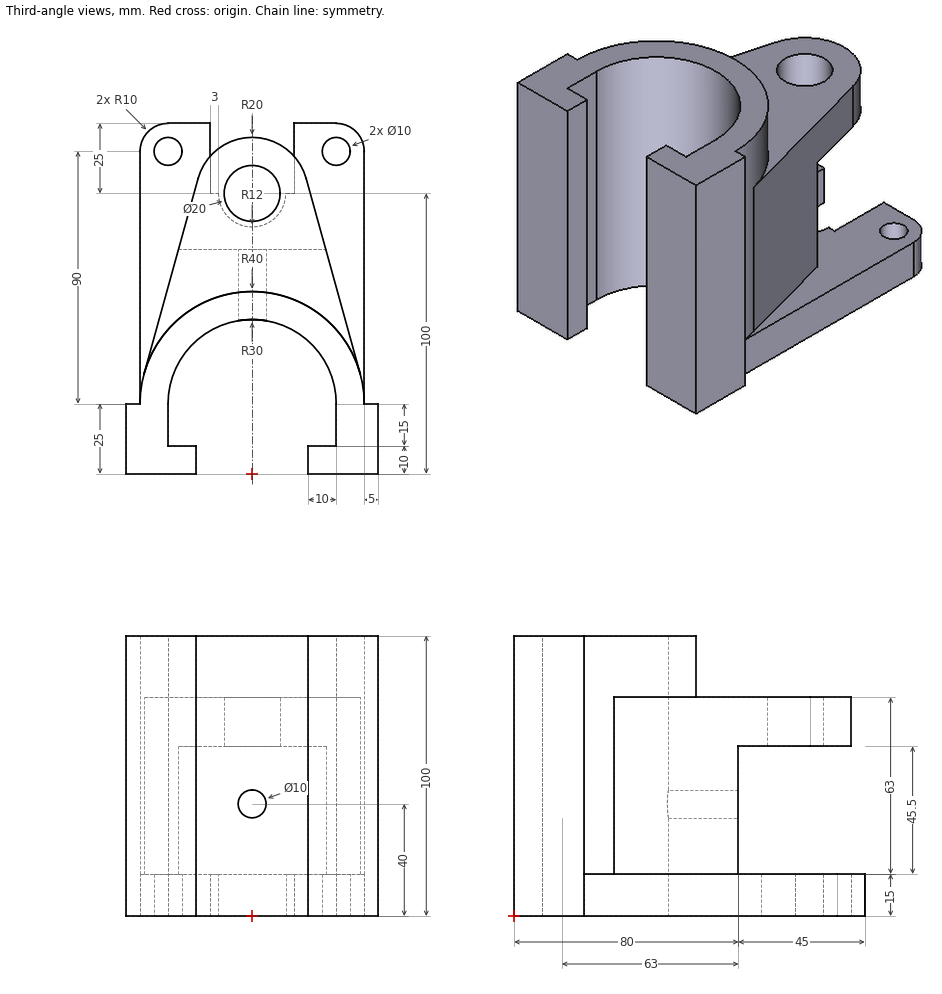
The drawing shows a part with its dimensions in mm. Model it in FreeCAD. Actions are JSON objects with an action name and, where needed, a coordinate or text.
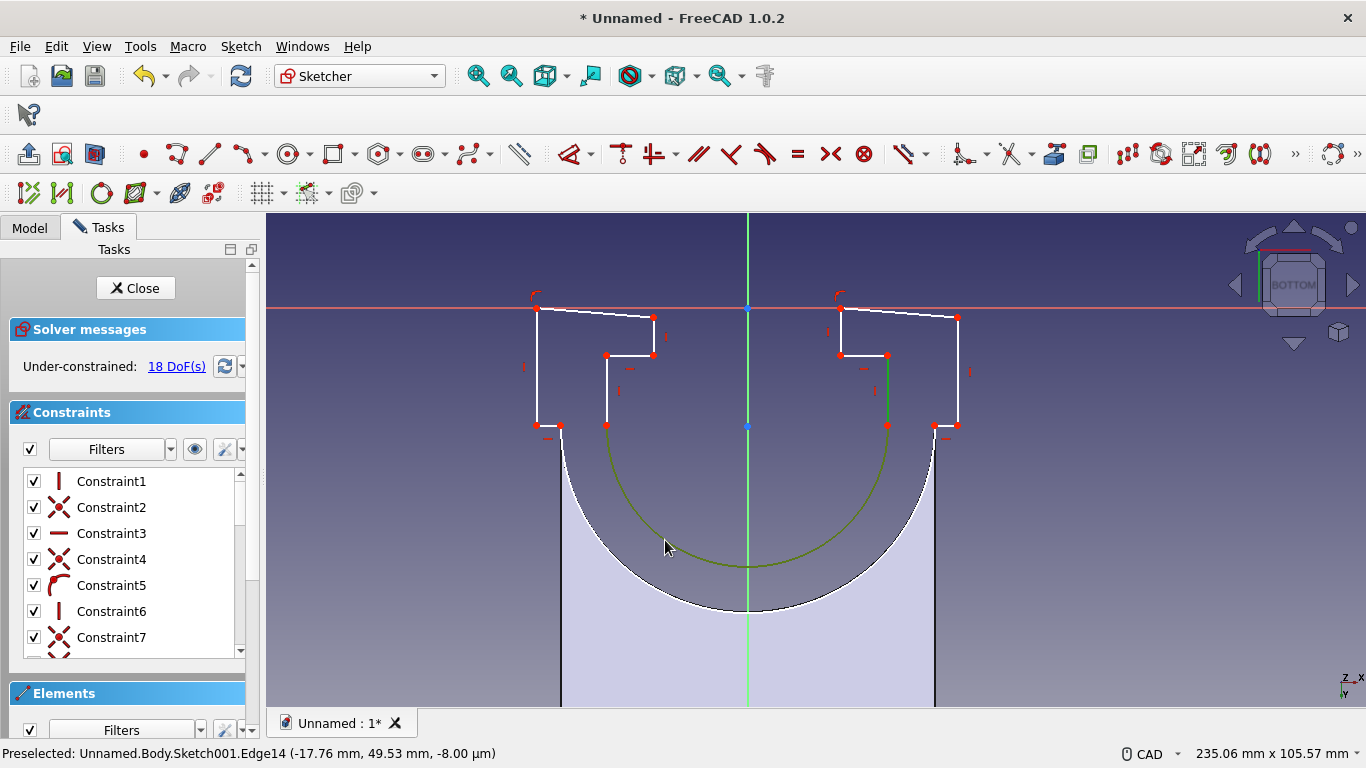
{"action": "key", "text": "t"}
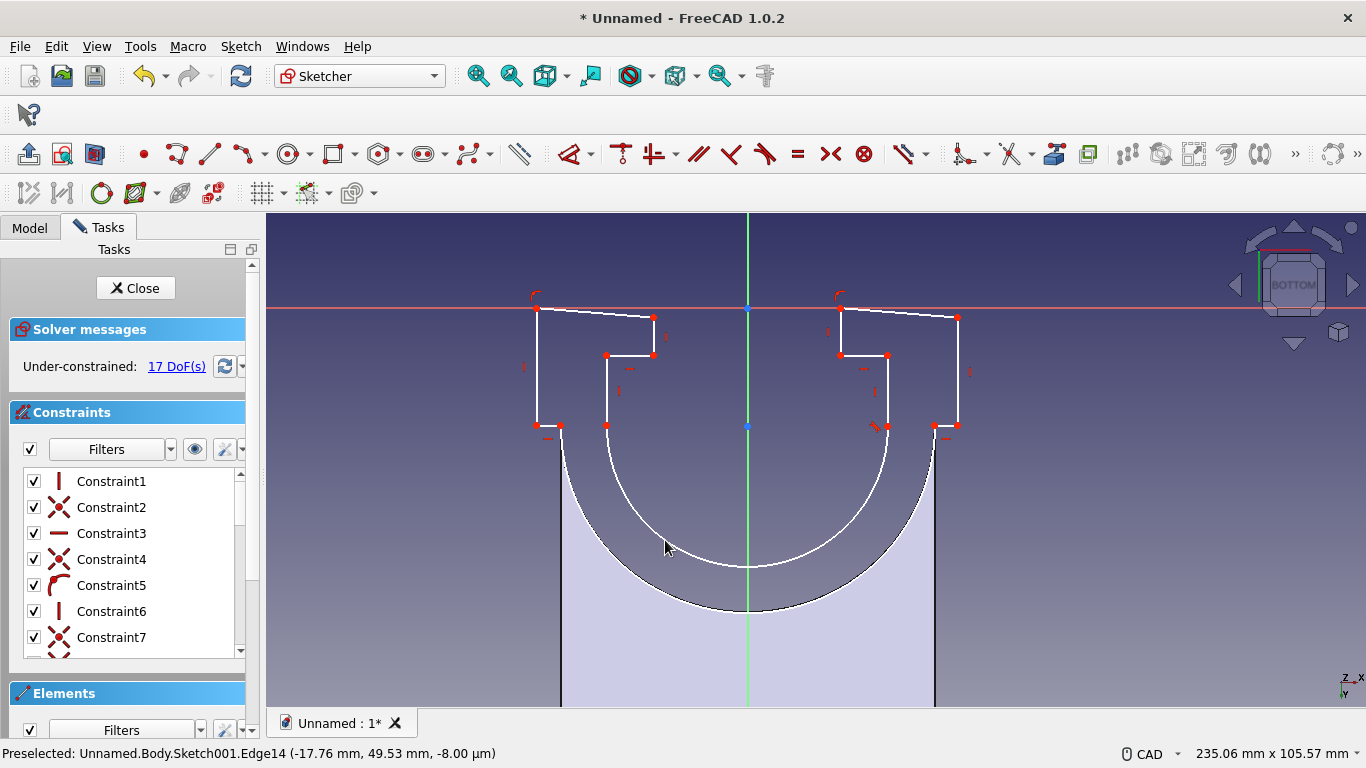
{"action": "left_click", "coordinate": [607, 377]}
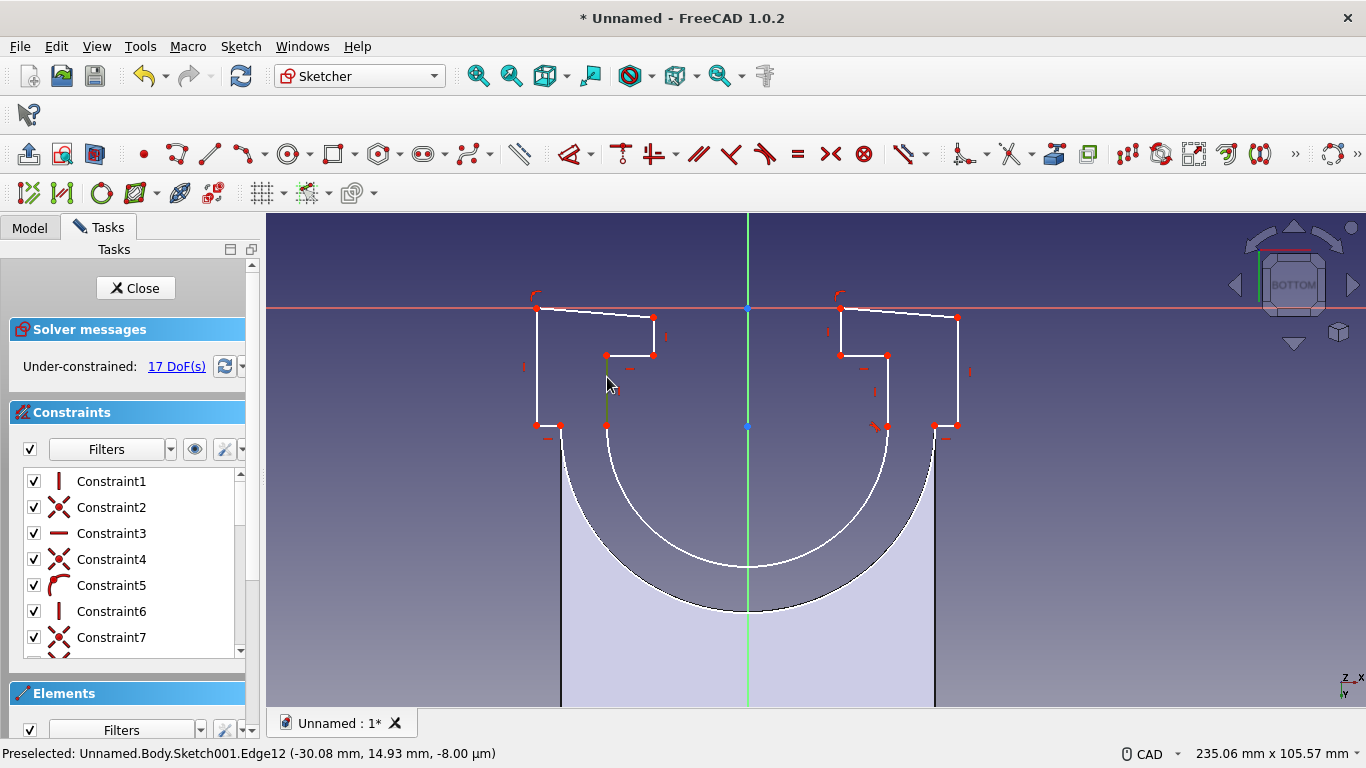
{"action": "left_click", "coordinate": [664, 540]}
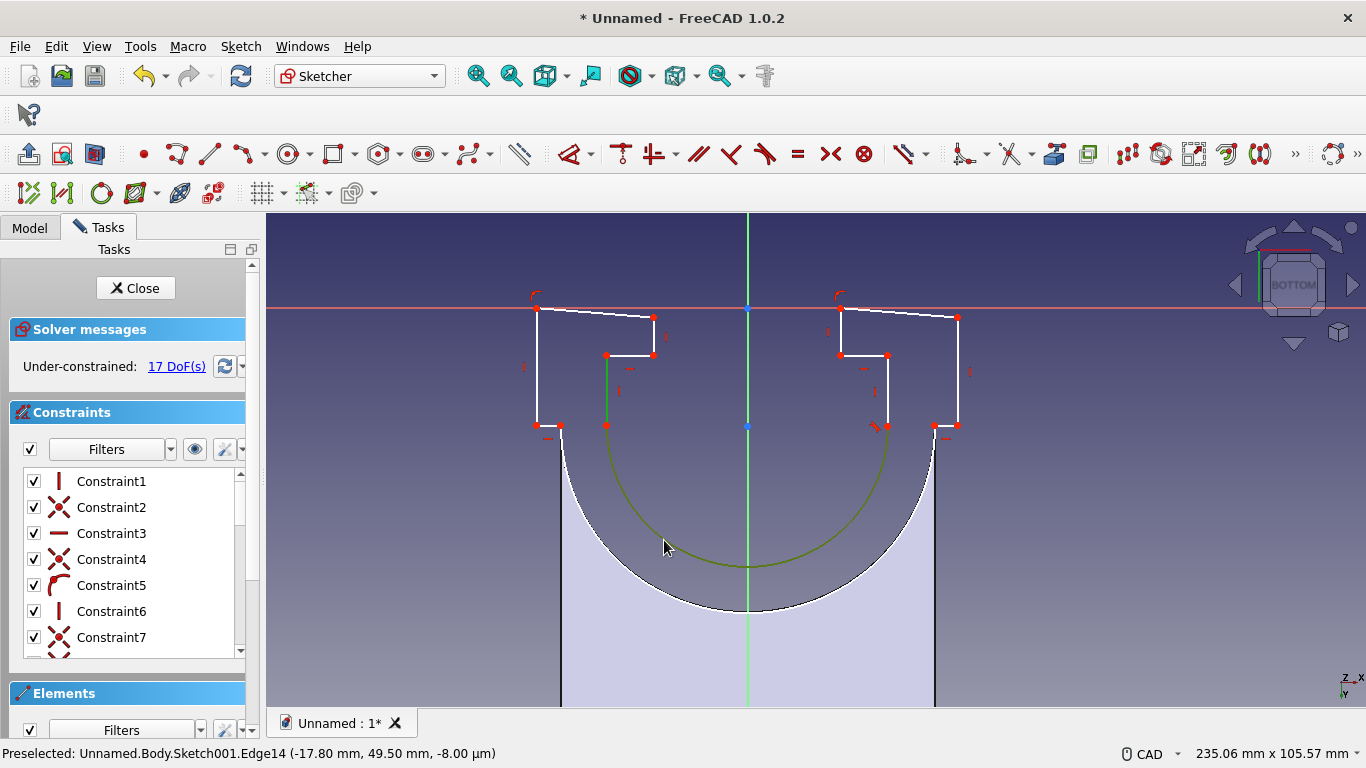
{"action": "key", "text": "t"}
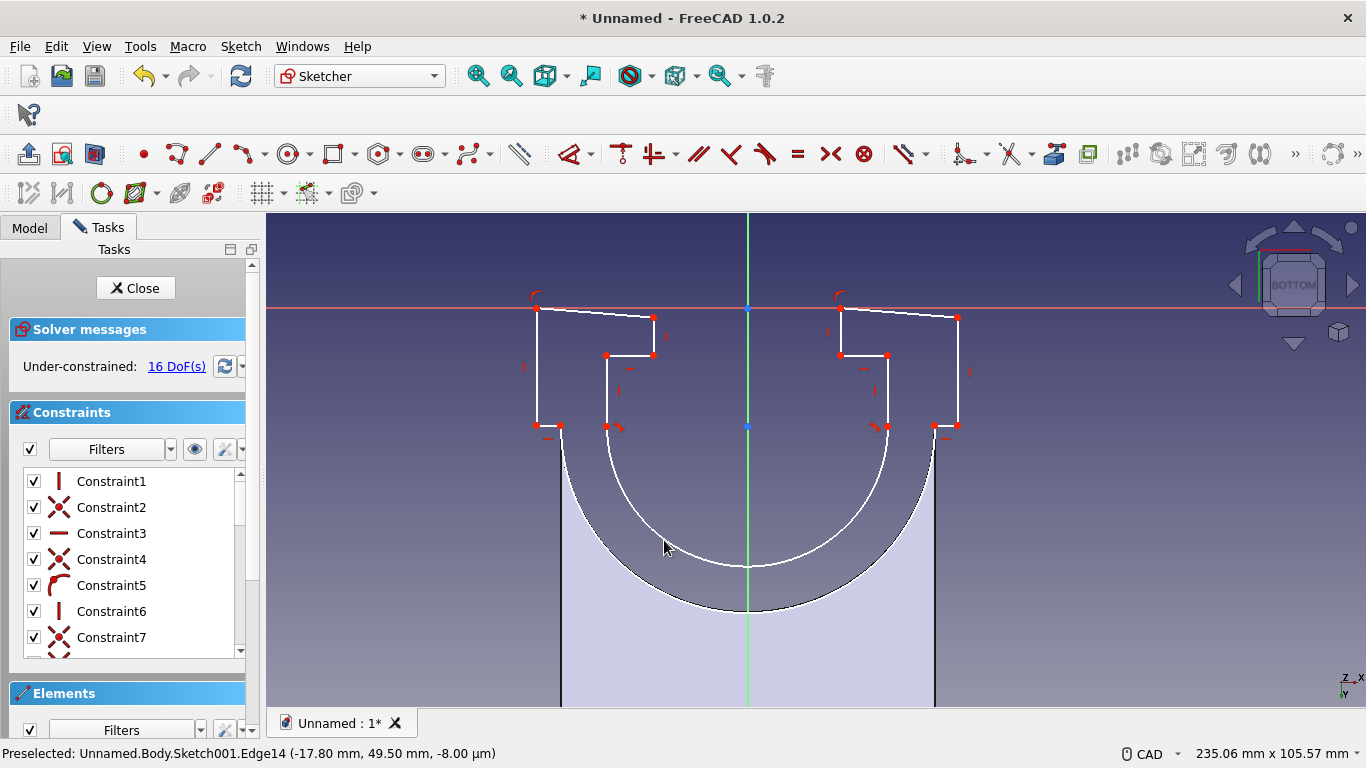
{"action": "left_click", "coordinate": [876, 311]}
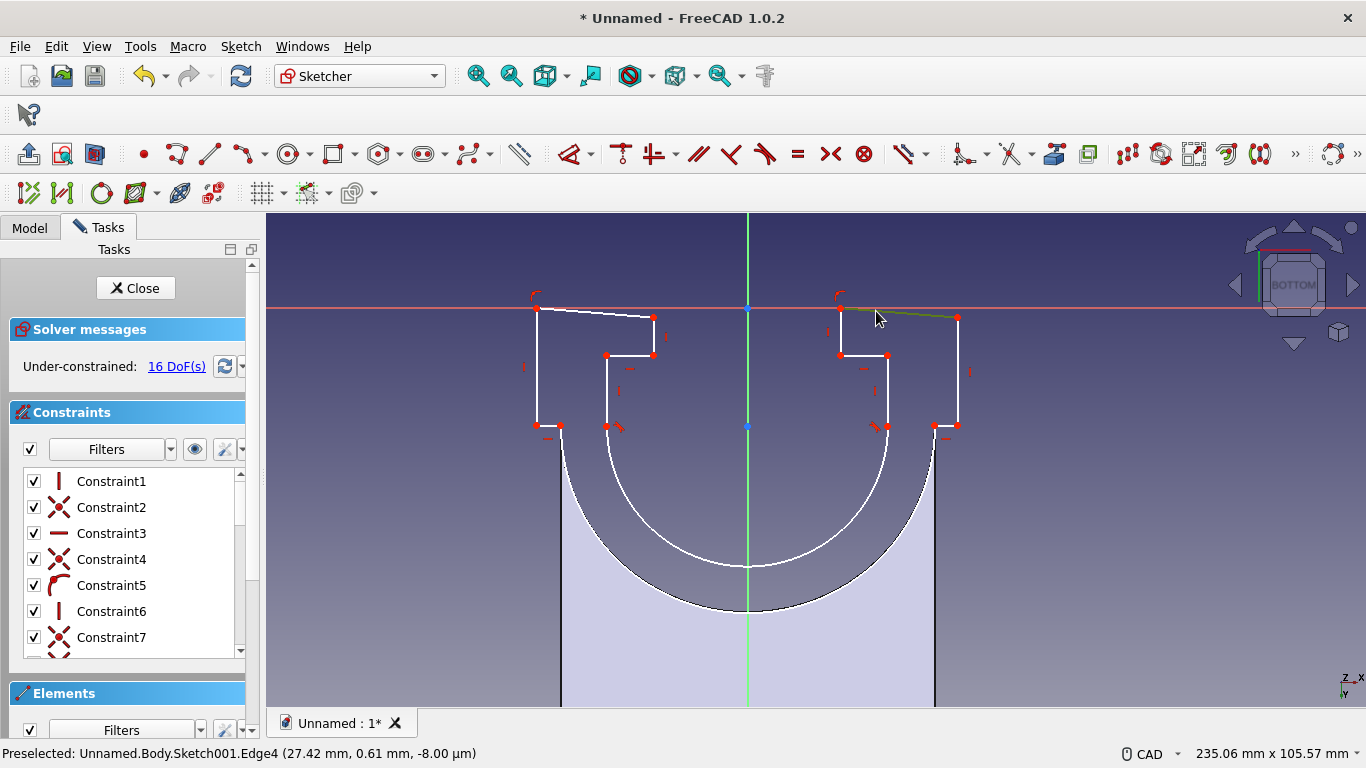
{"action": "key", "text": "h"}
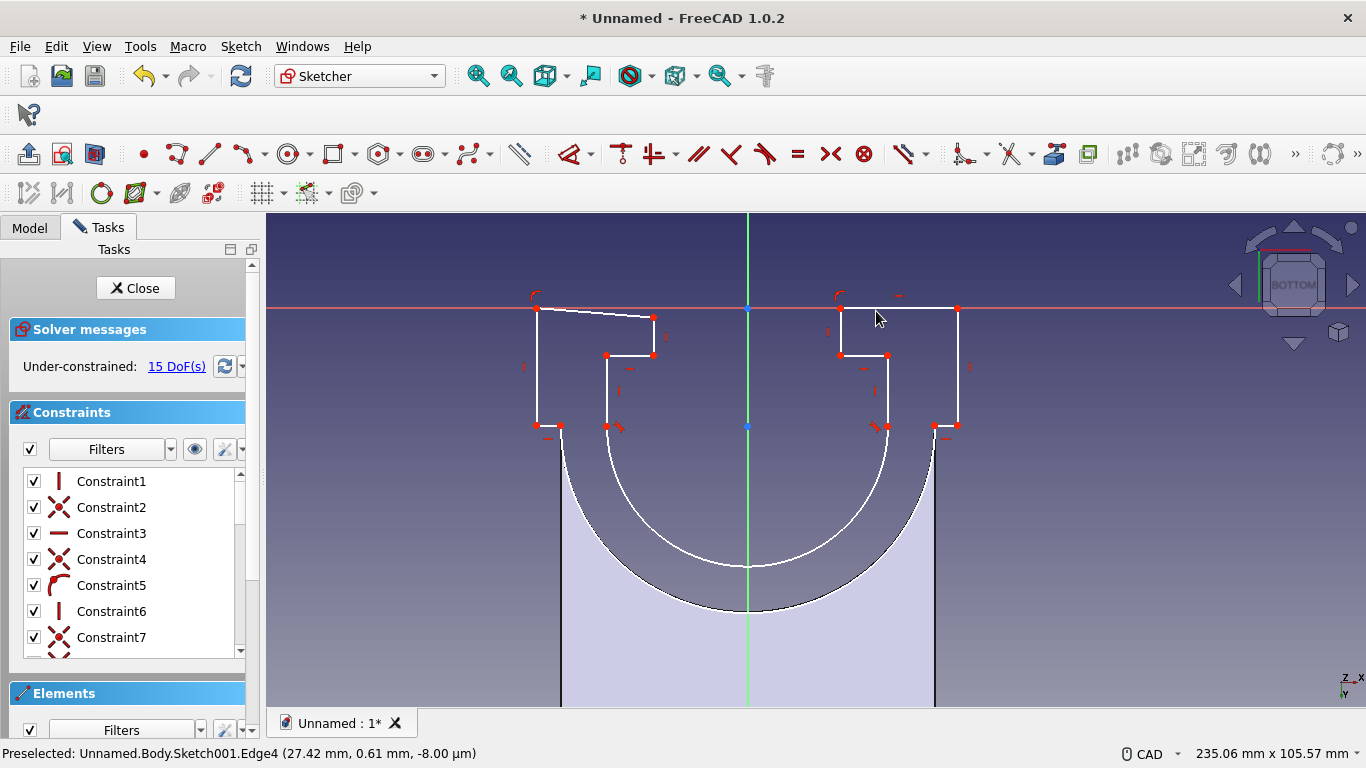
{"action": "left_click", "coordinate": [572, 311]}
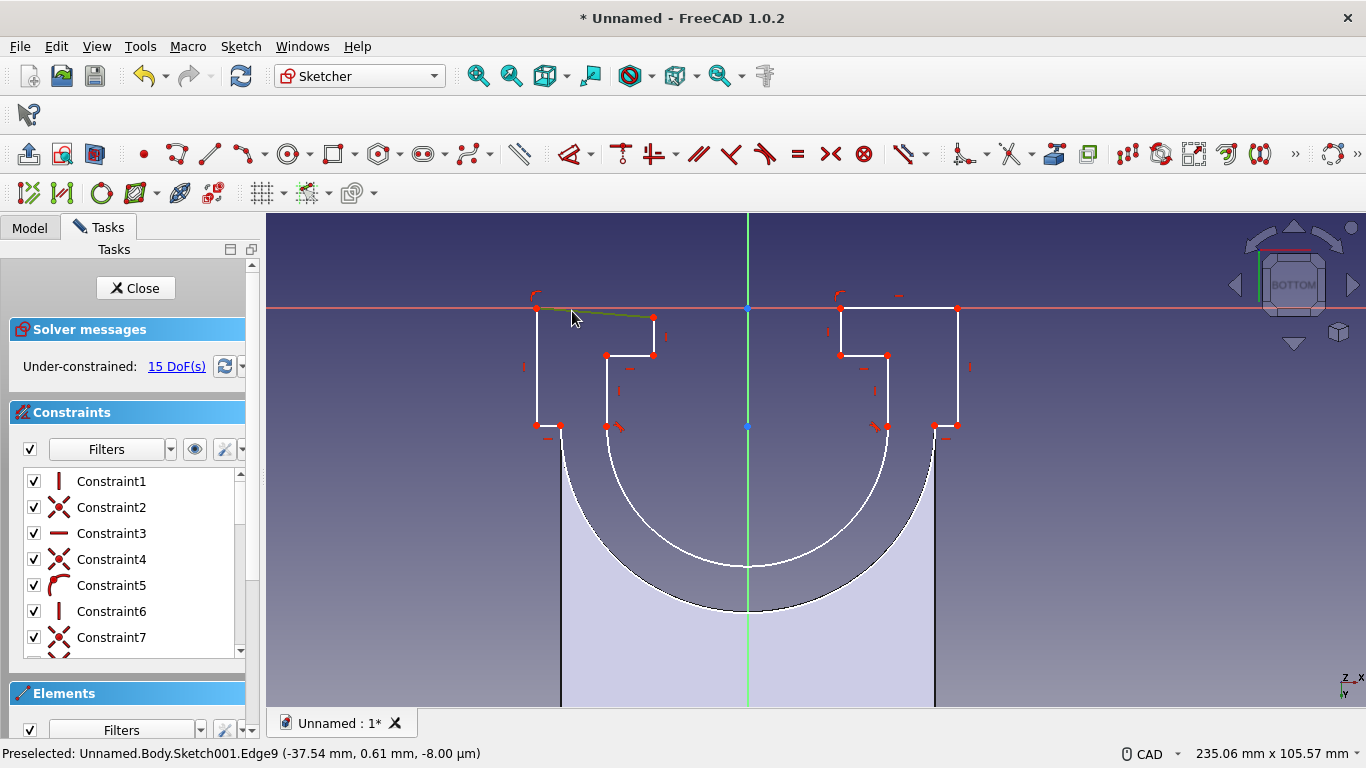
{"action": "key", "text": "h"}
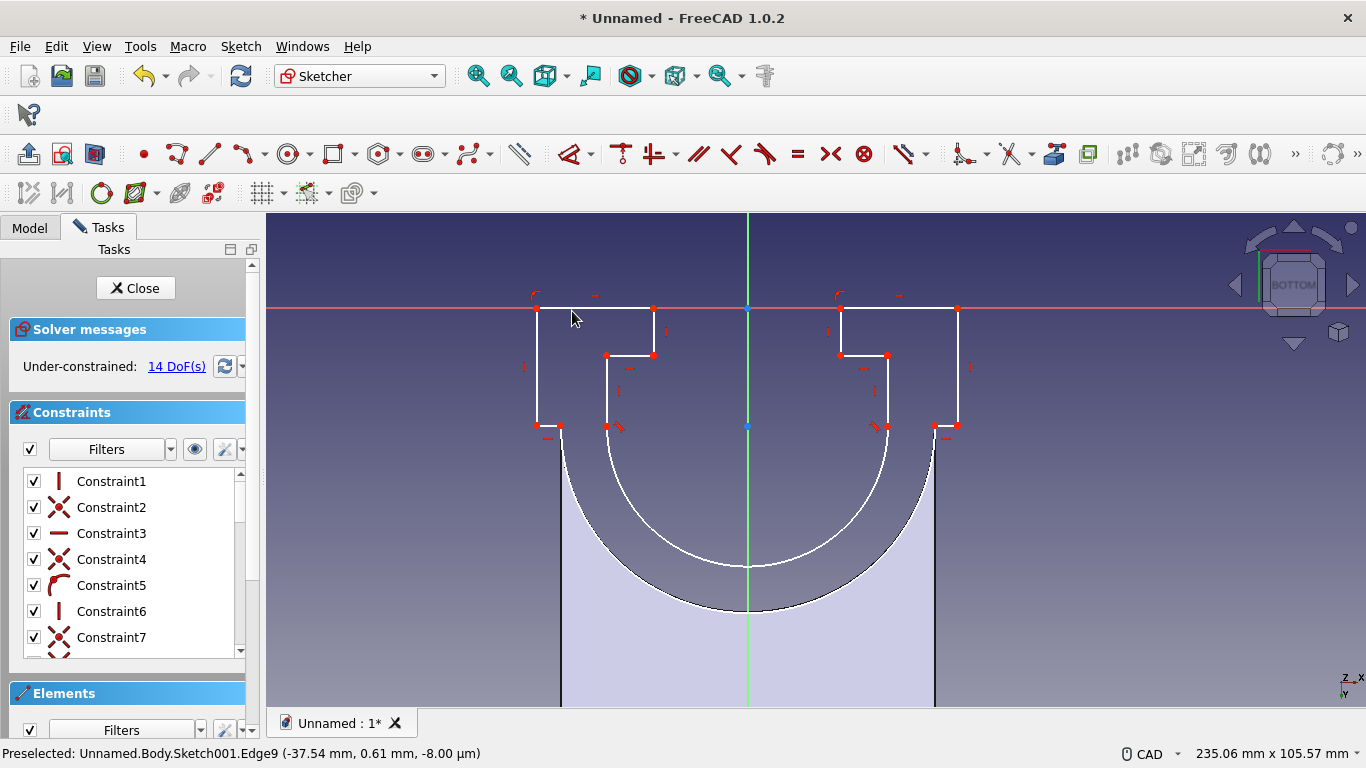
{"action": "left_click", "coordinate": [638, 577]}